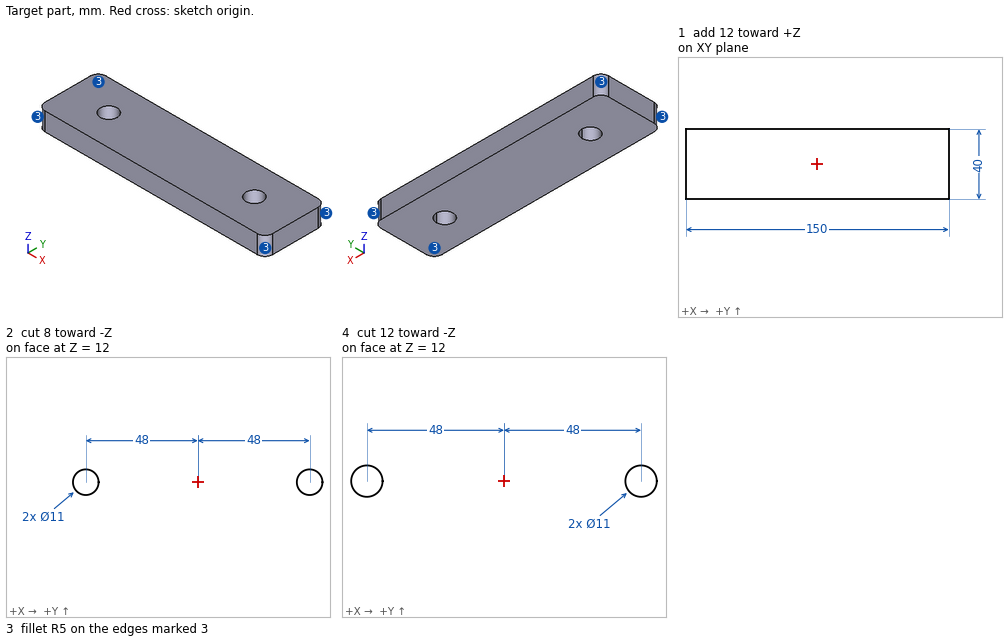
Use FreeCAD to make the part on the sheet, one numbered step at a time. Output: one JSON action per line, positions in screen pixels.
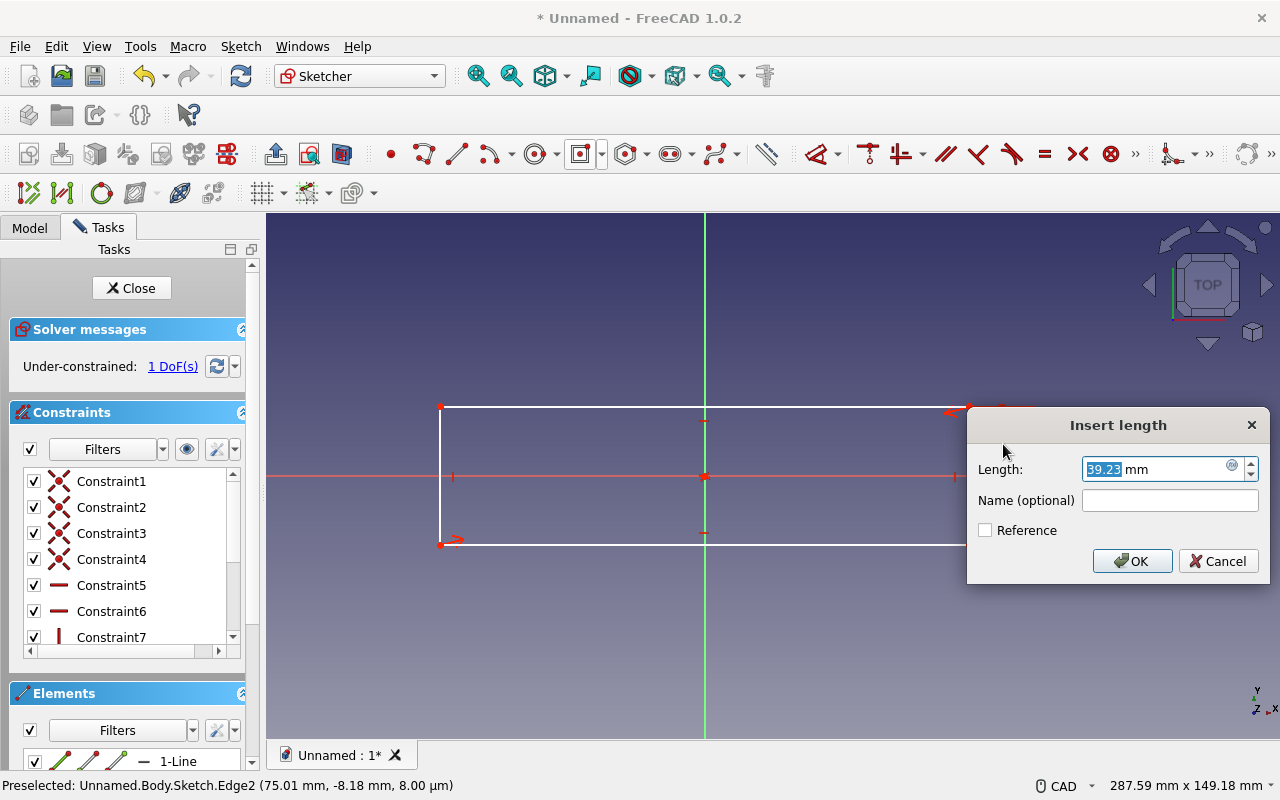
{"action": "type", "text": "40"}
{"action": "key", "text": "Return"}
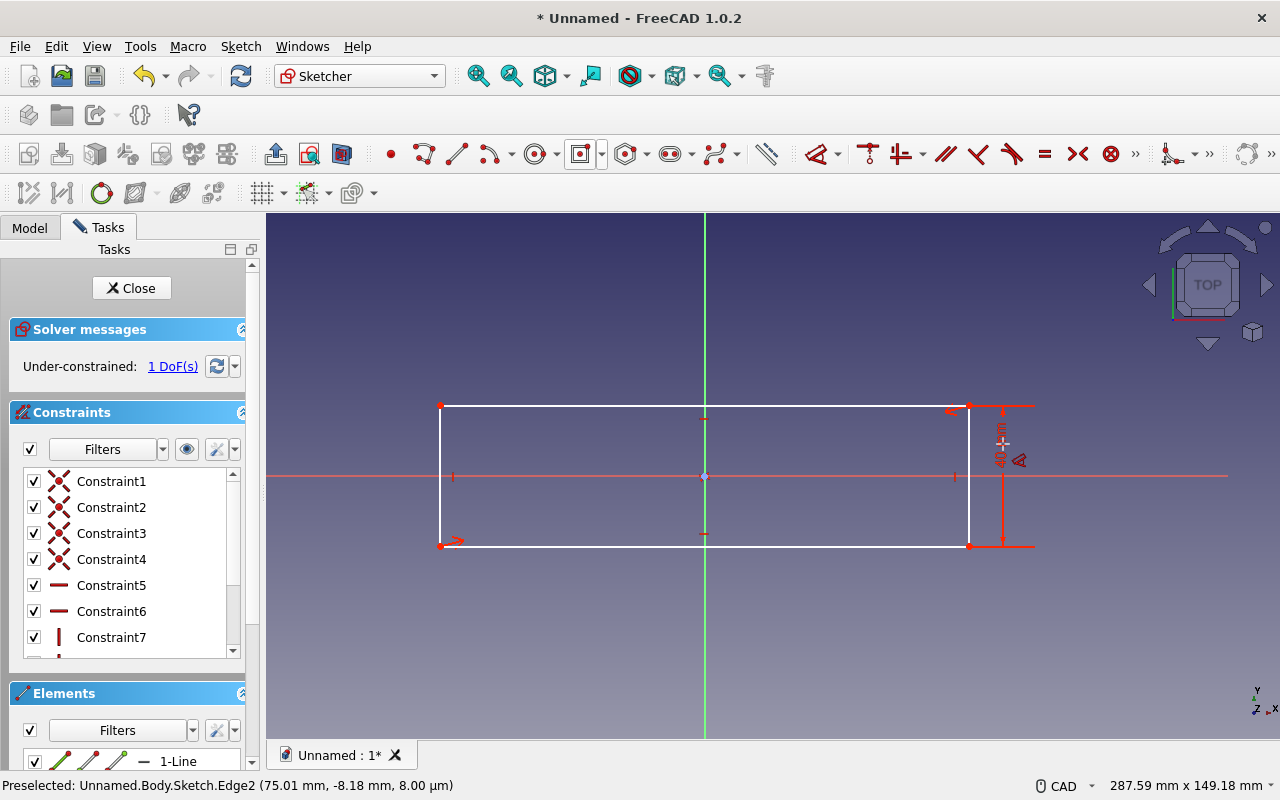
{"action": "left_click", "coordinate": [599, 547]}
{"action": "left_click", "coordinate": [583, 581]}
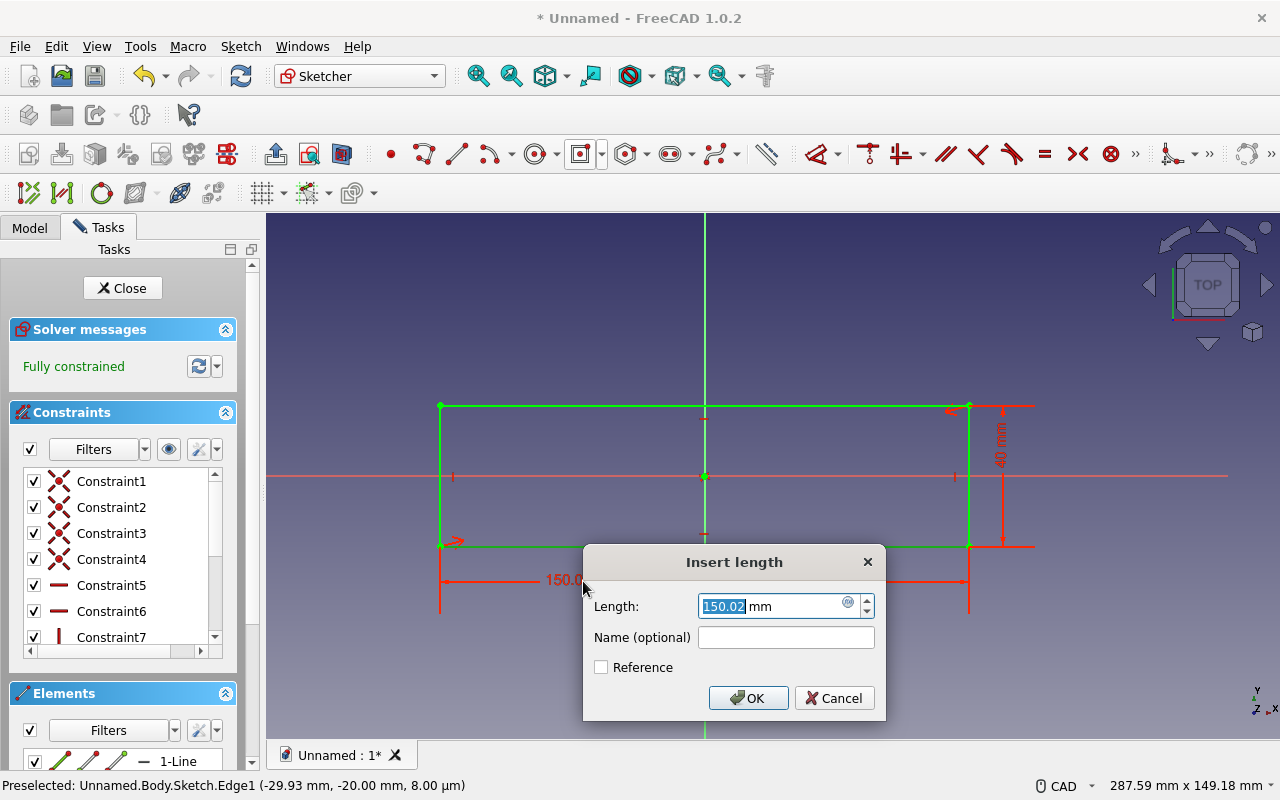
{"action": "type", "text": "150"}
{"action": "key", "text": "Return"}
{"action": "key", "text": "Escape"}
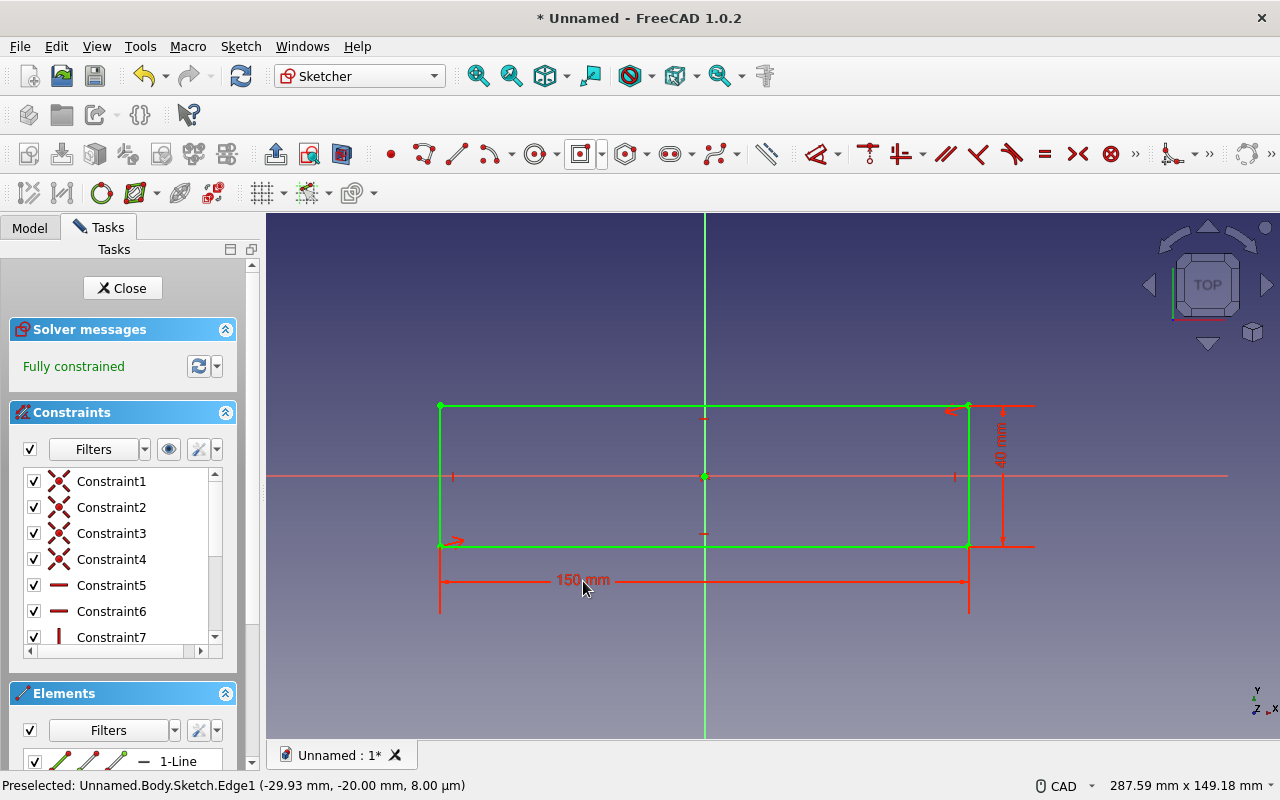
{"action": "left_click", "coordinate": [123, 288]}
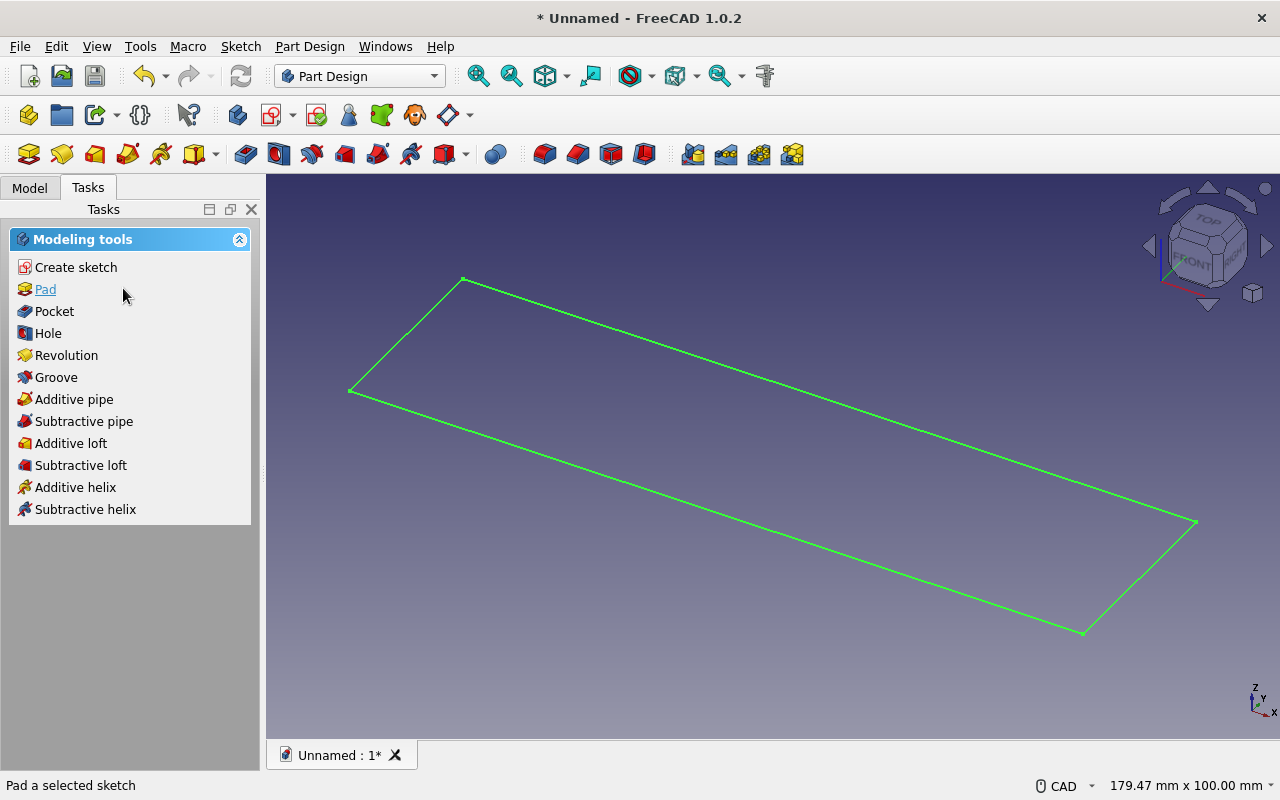
{"action": "left_click", "coordinate": [29, 154]}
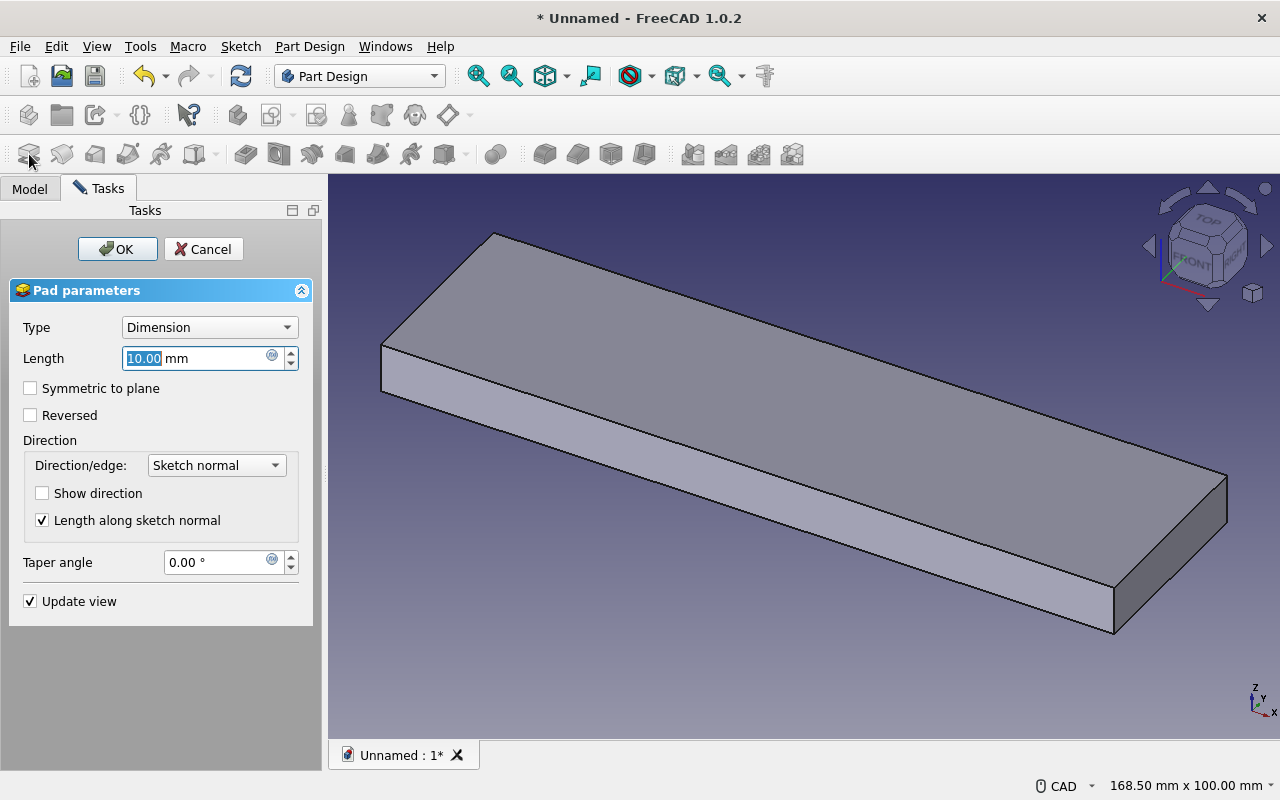
{"action": "type", "text": "12"}
{"action": "key", "text": "Tab"}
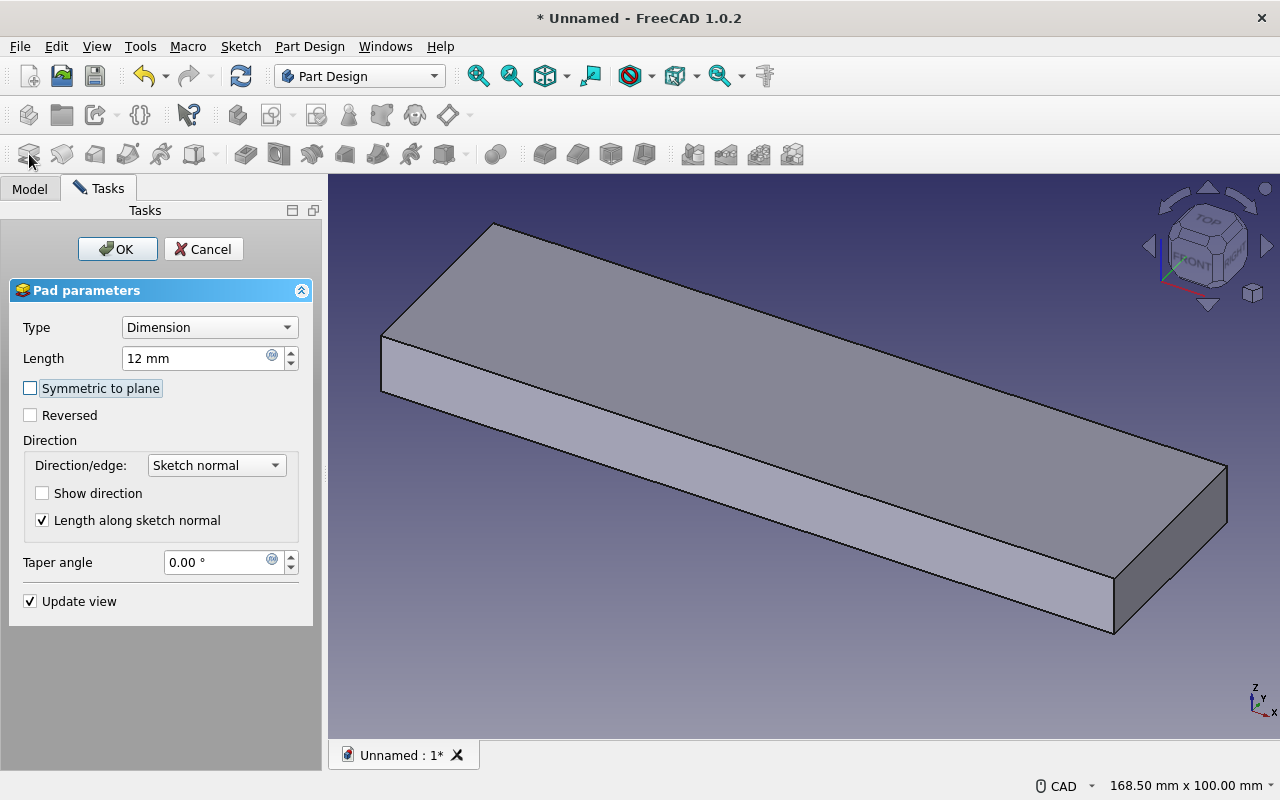
{"action": "left_click", "coordinate": [118, 249]}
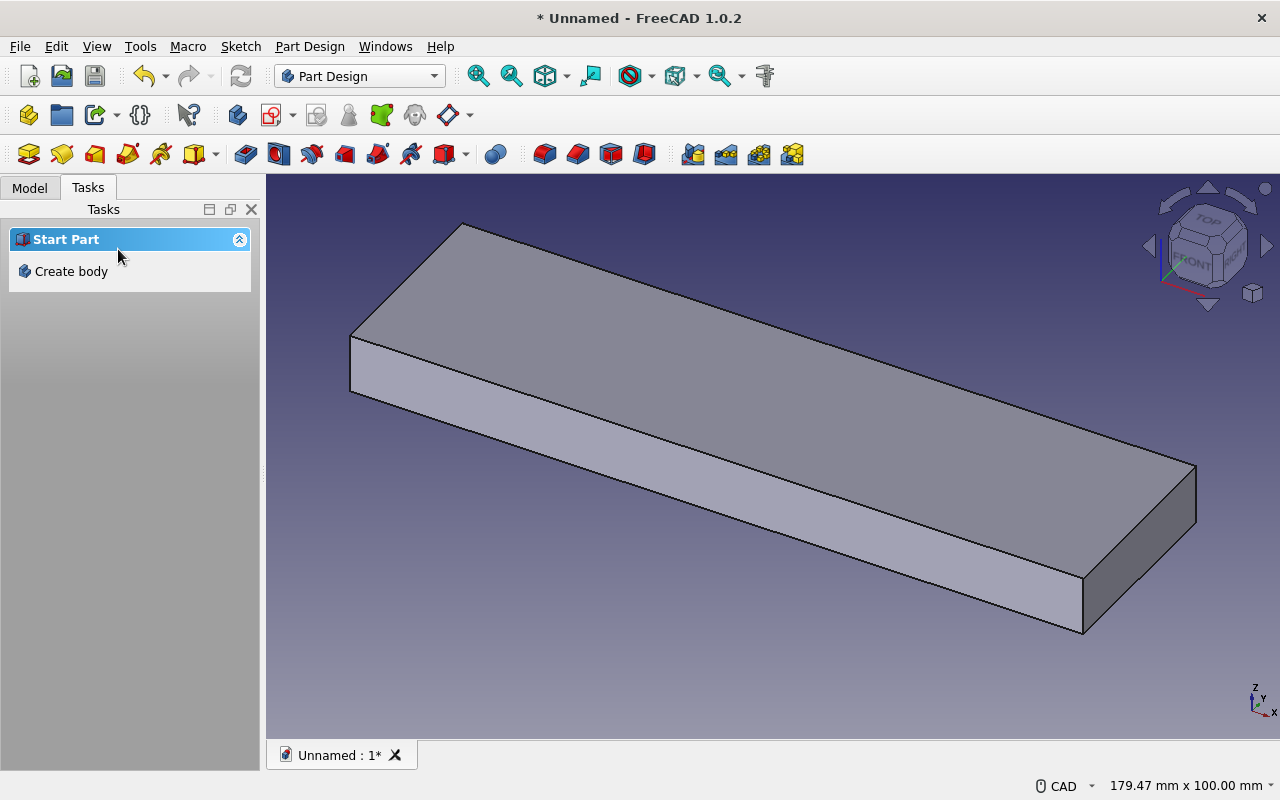
{"action": "left_click", "coordinate": [983, 469]}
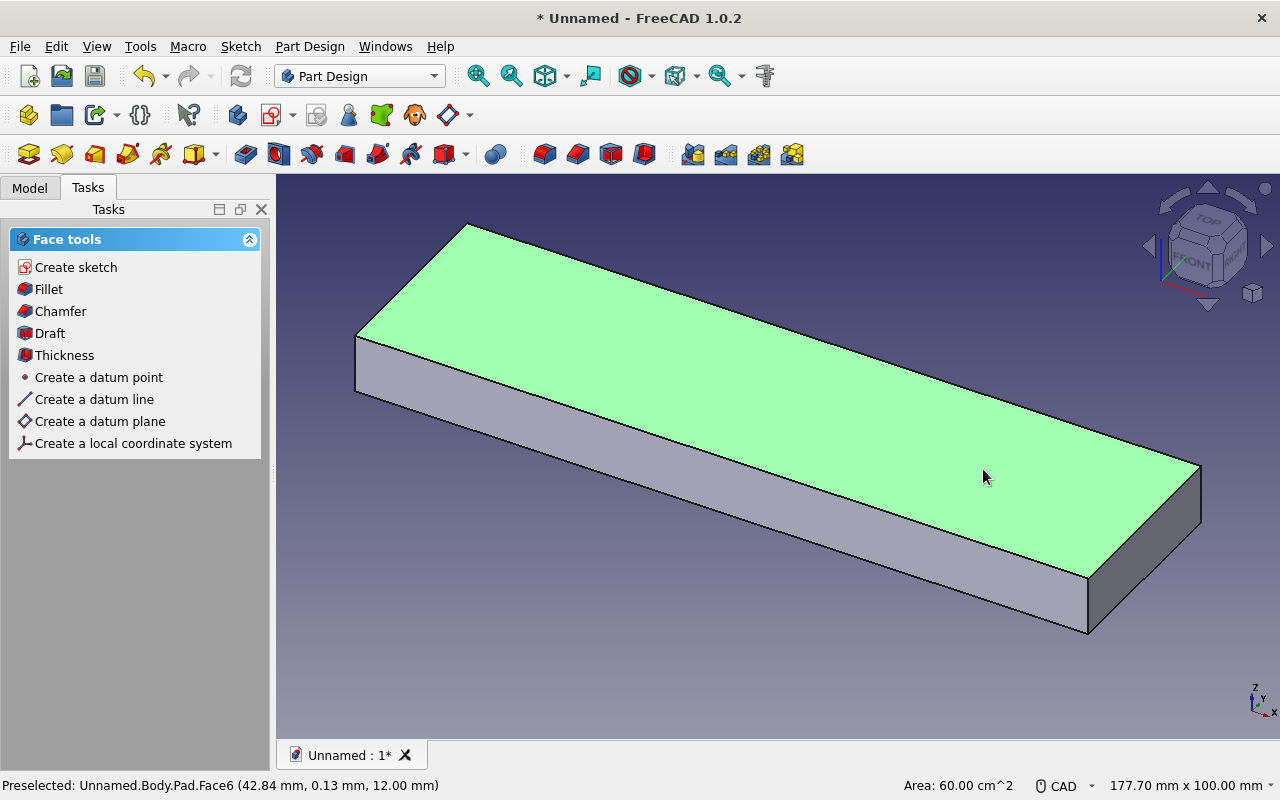
{"action": "left_click", "coordinate": [270, 116]}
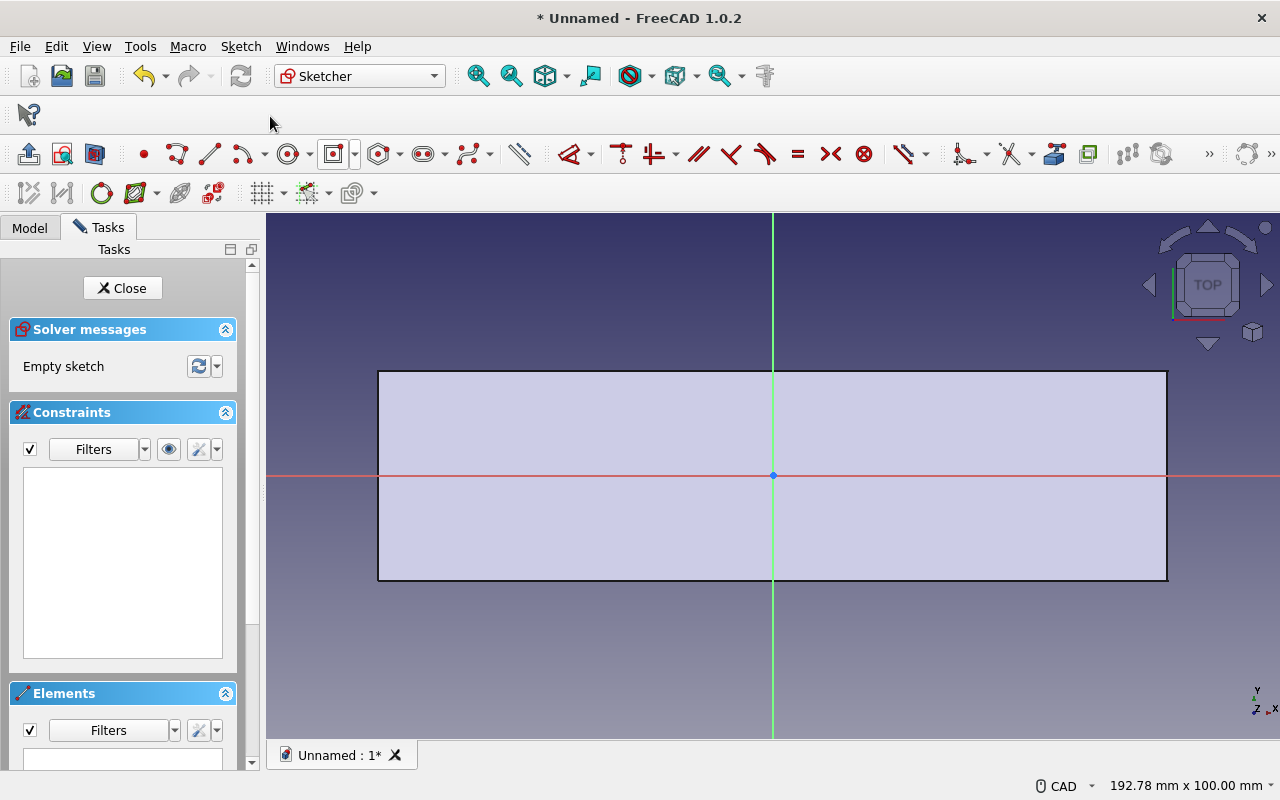
{"action": "left_click", "coordinate": [288, 154]}